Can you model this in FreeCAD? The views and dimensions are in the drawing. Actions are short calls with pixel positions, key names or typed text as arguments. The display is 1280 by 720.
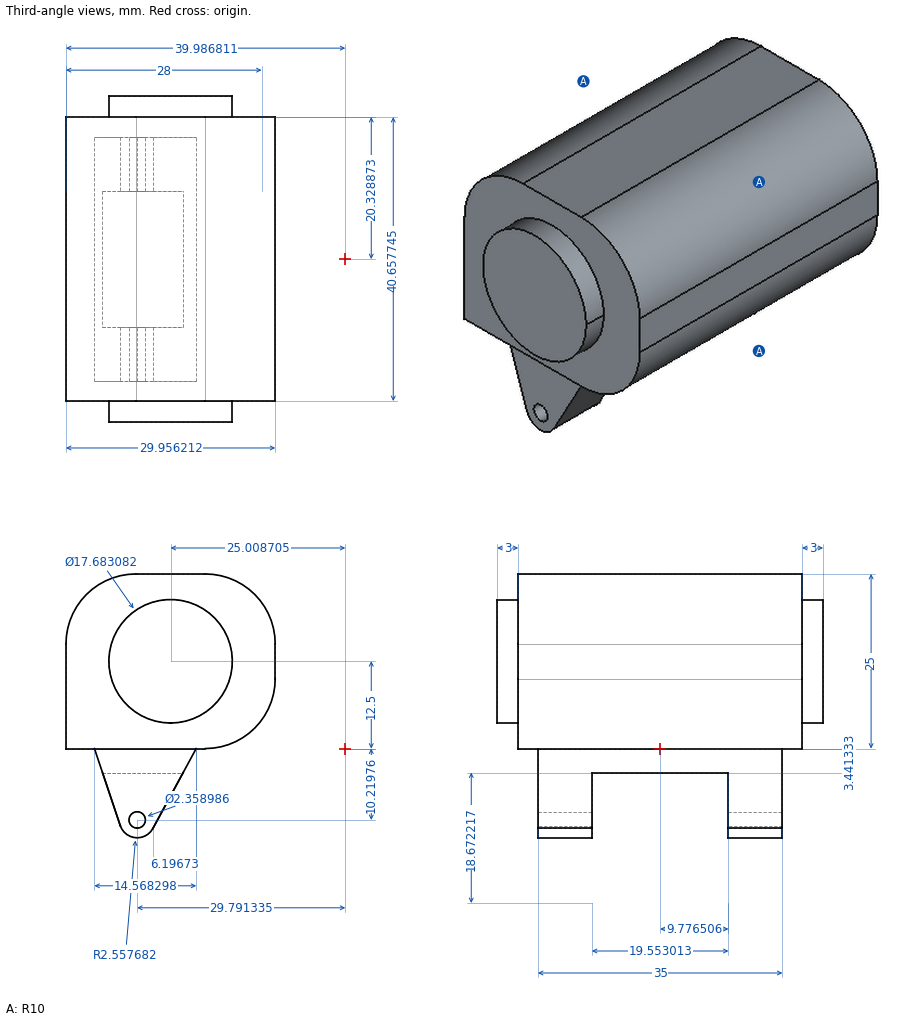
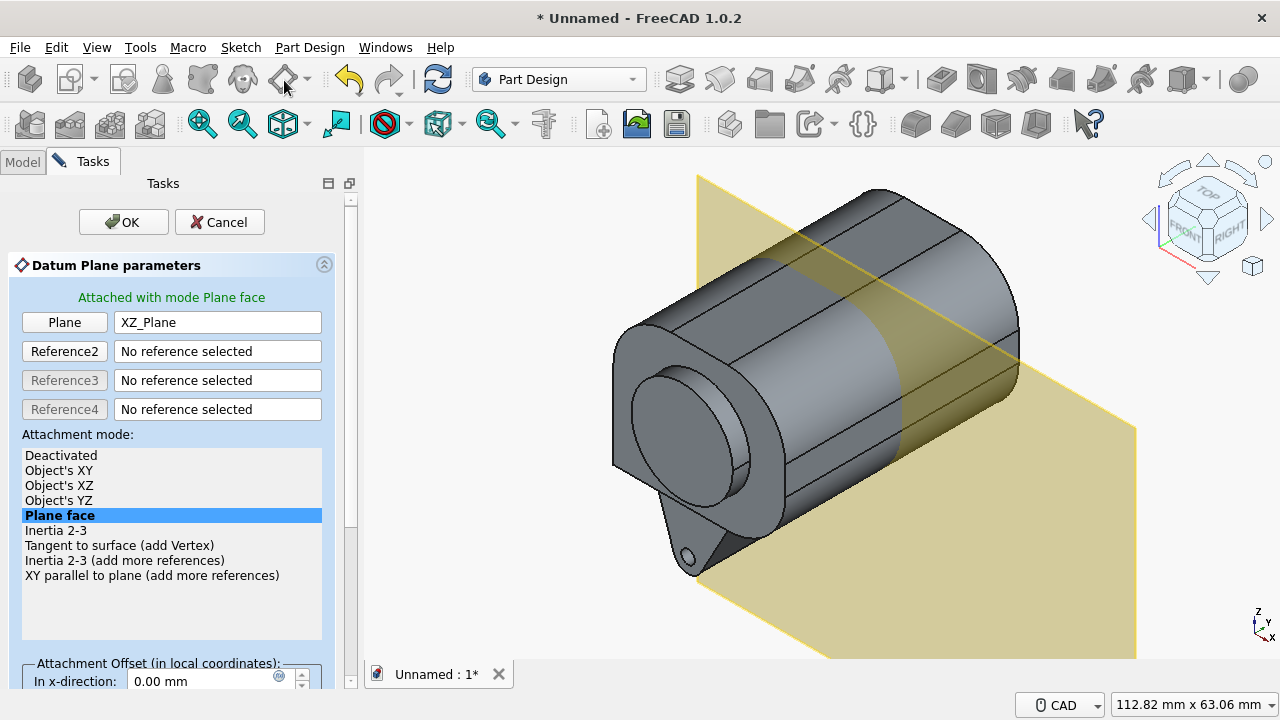
scroll(351, 440, down, 3)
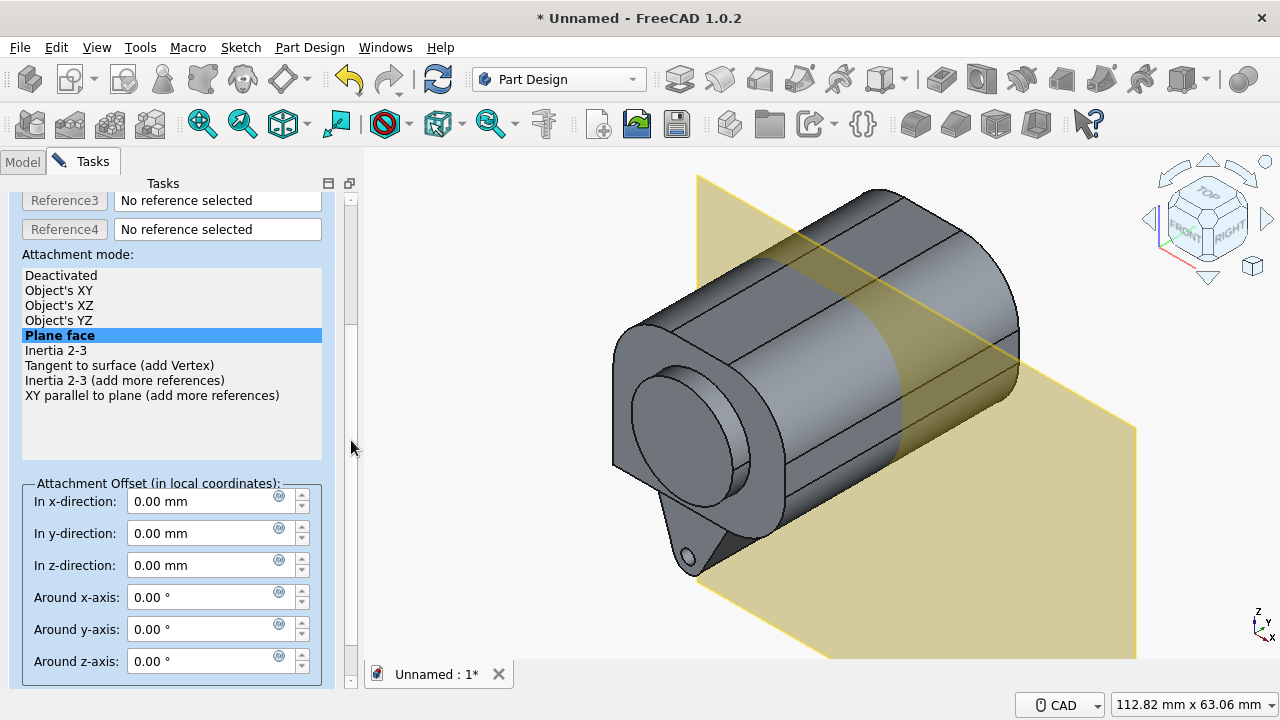
triple_click(210, 565)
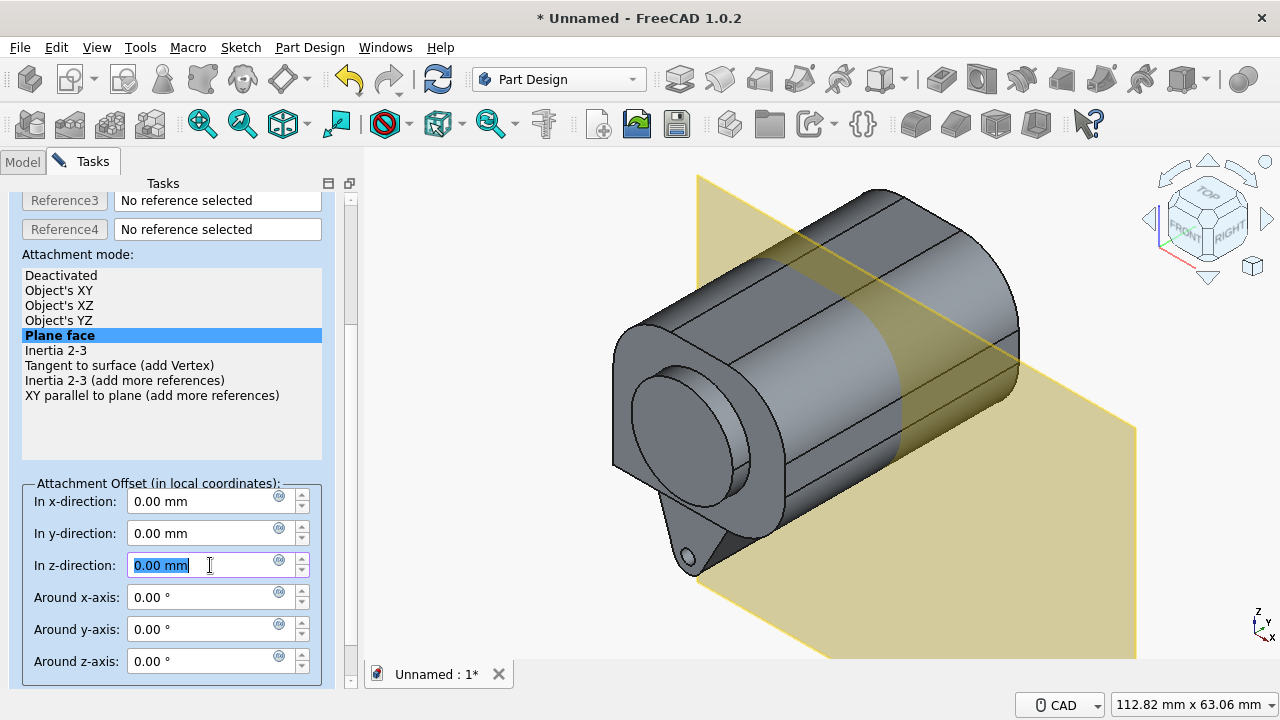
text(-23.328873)
key(Tab)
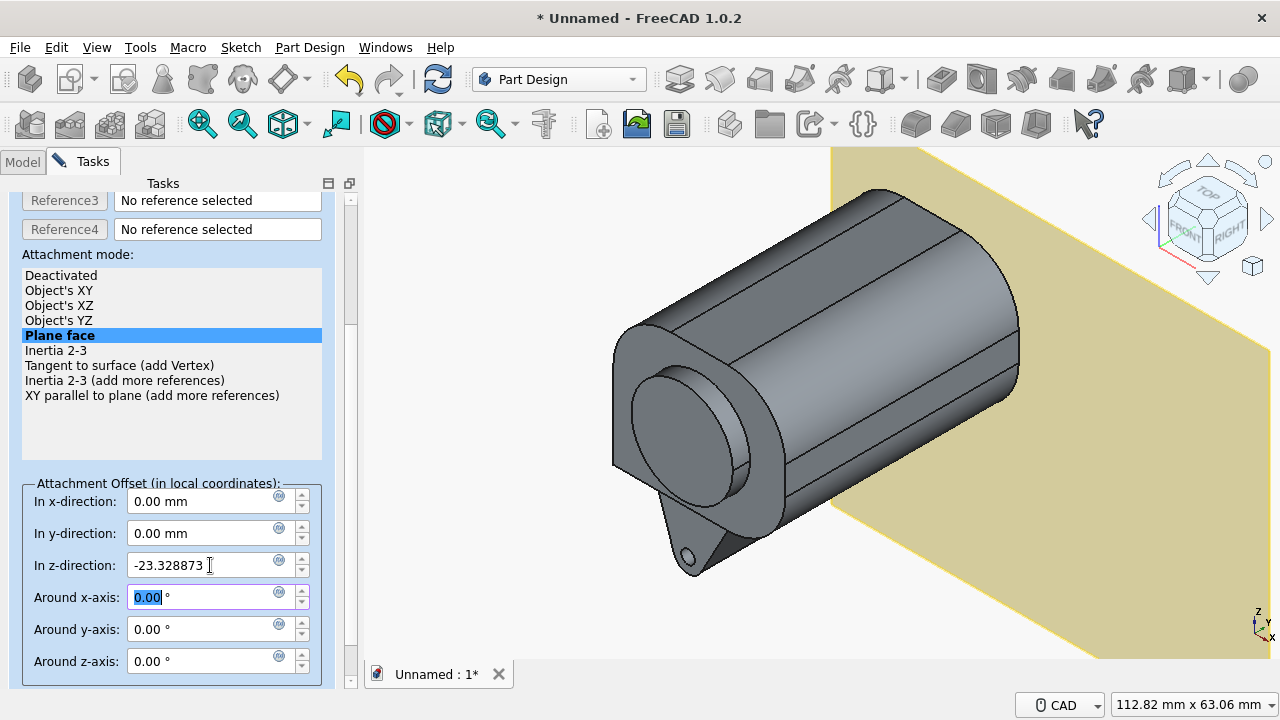
scroll(351, 440, up, 4)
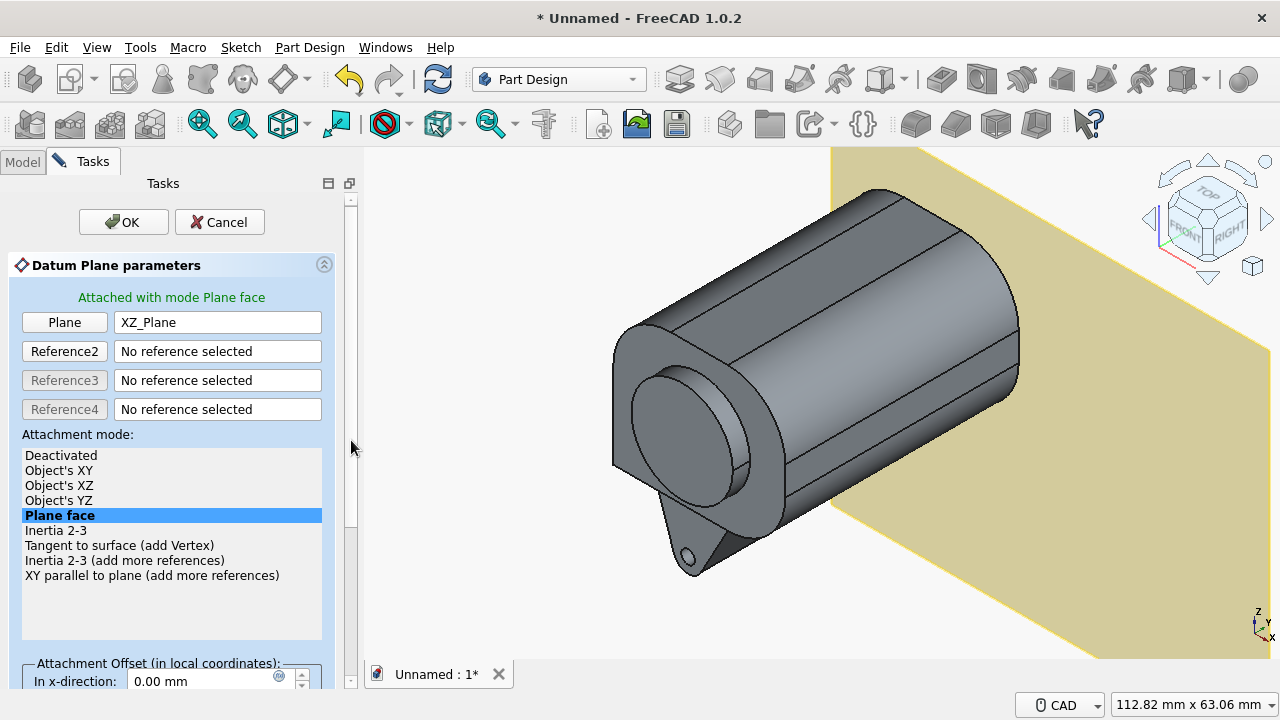
click(124, 222)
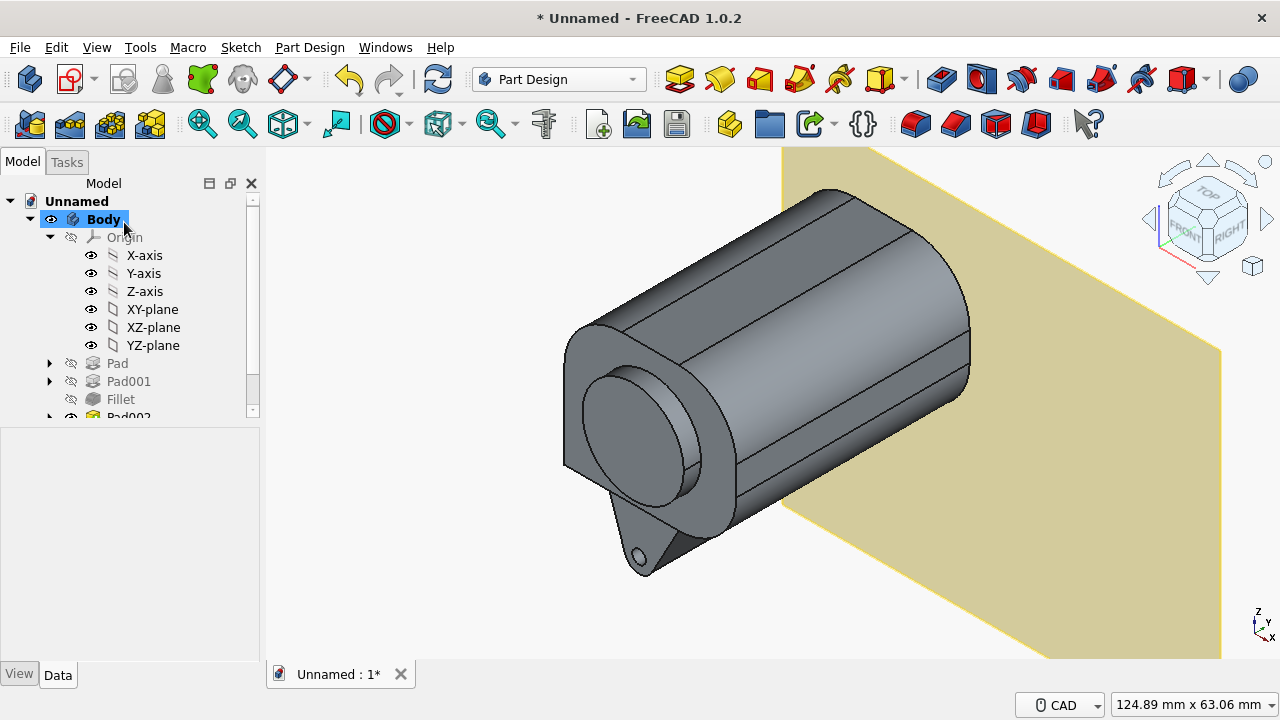
scroll(100, 305, down, 3)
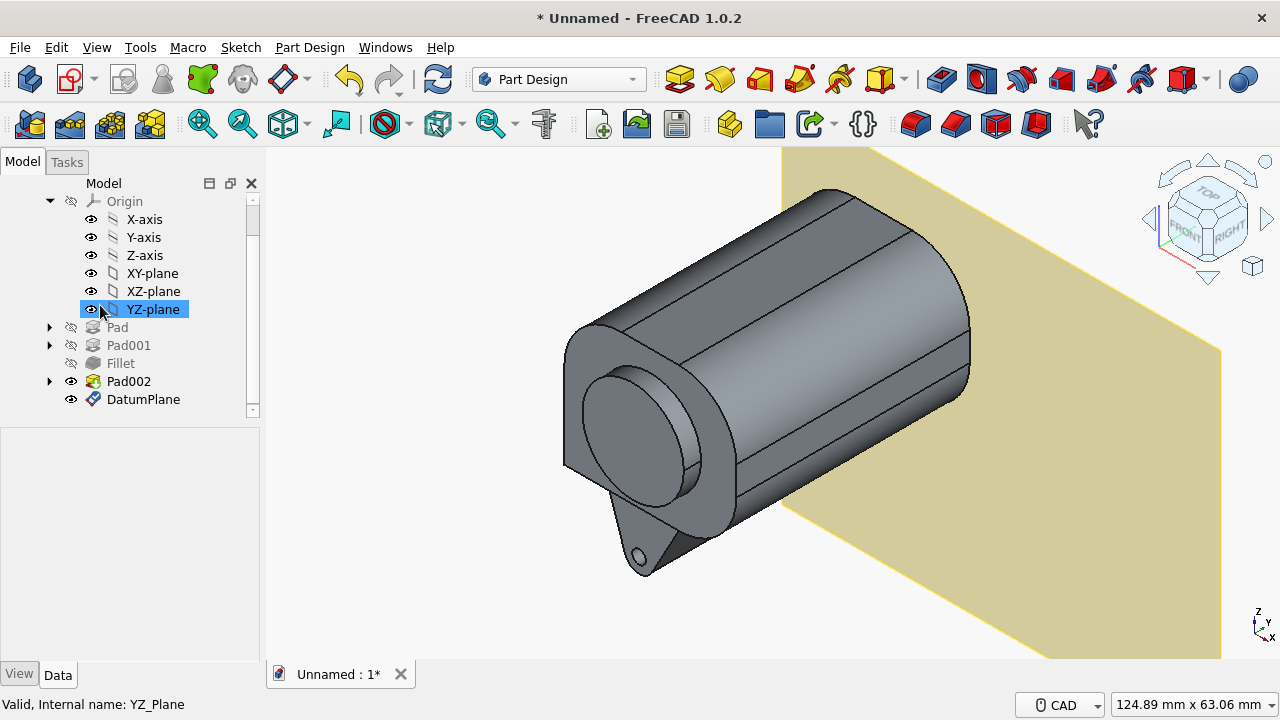
click(116, 399)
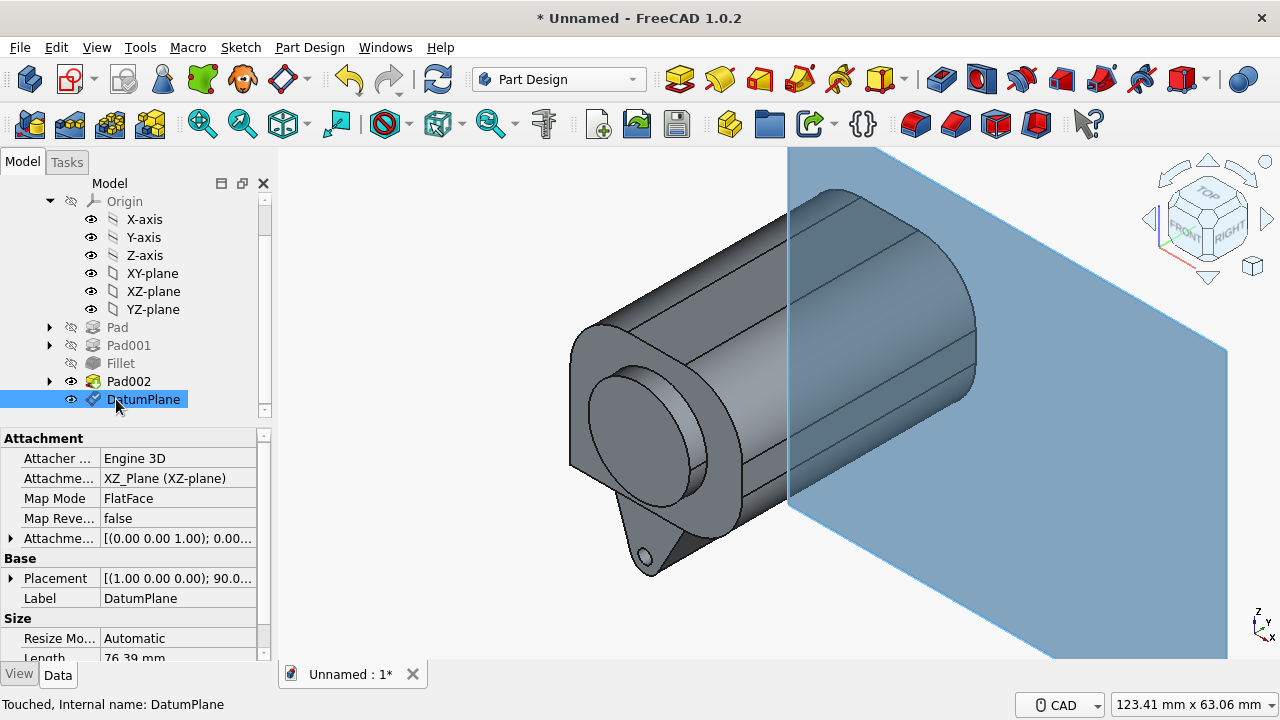
click(70, 80)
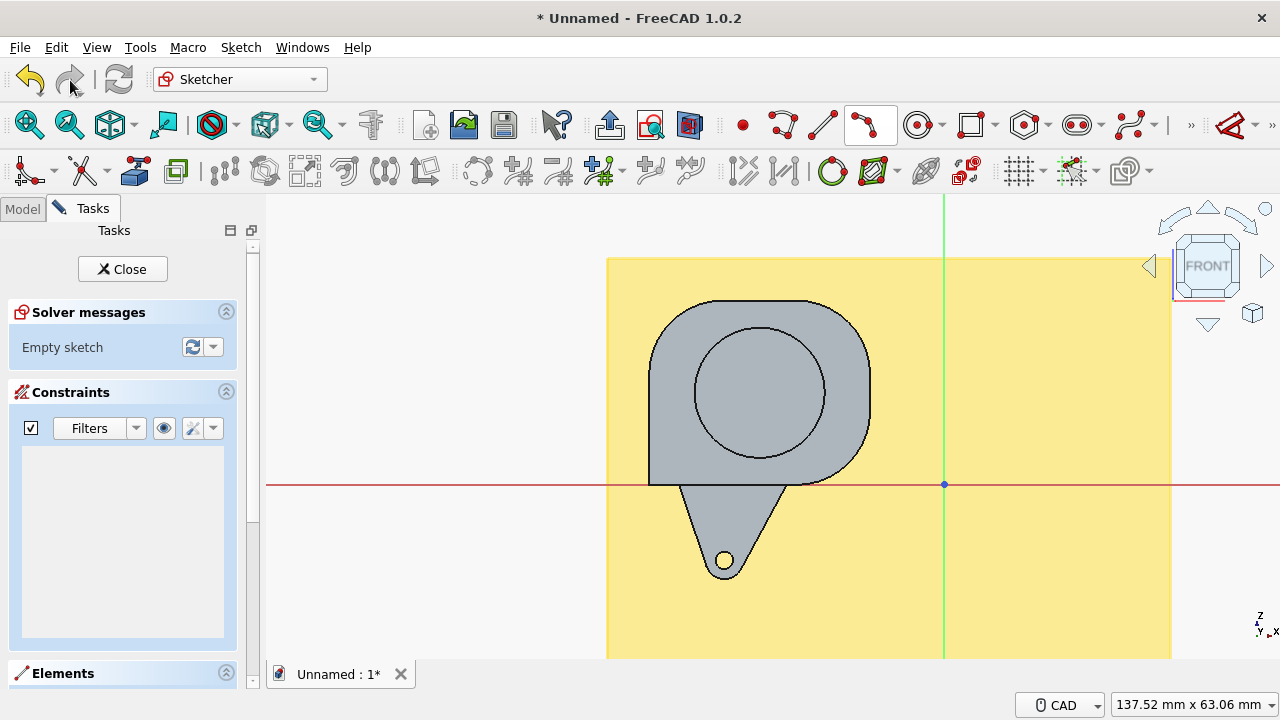
click(690, 126)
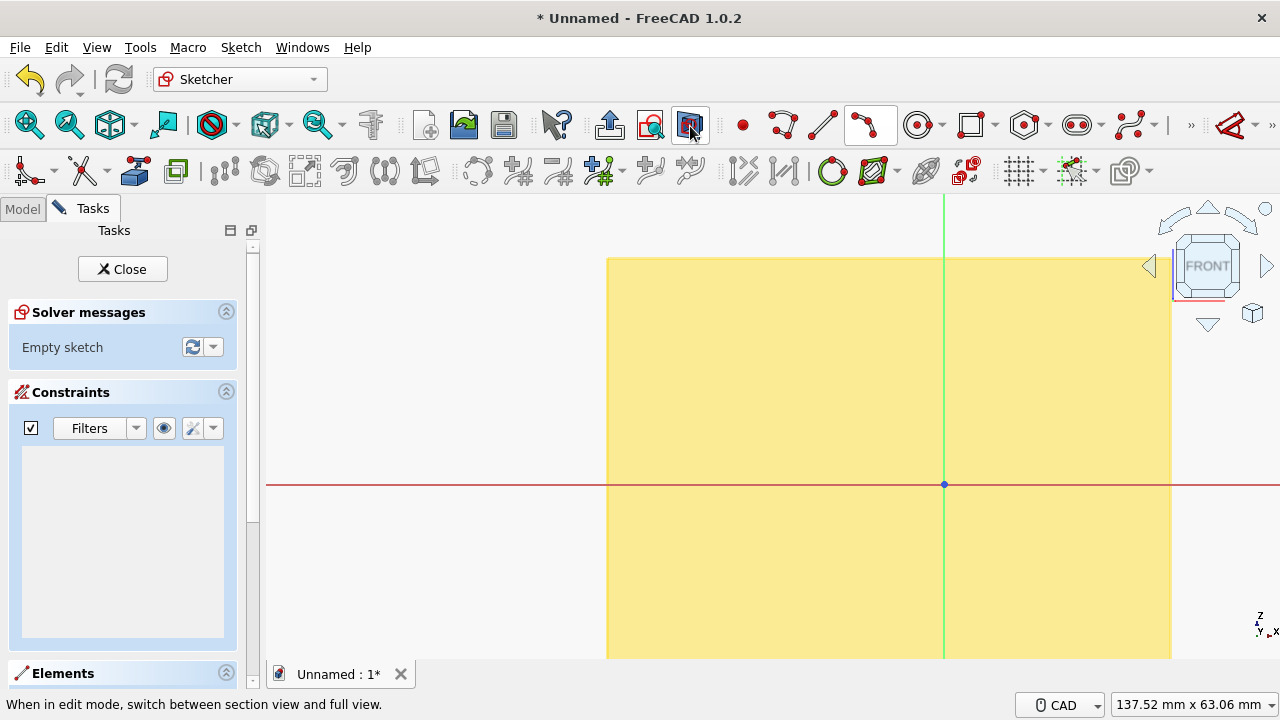
scroll(959, 382, up, 3)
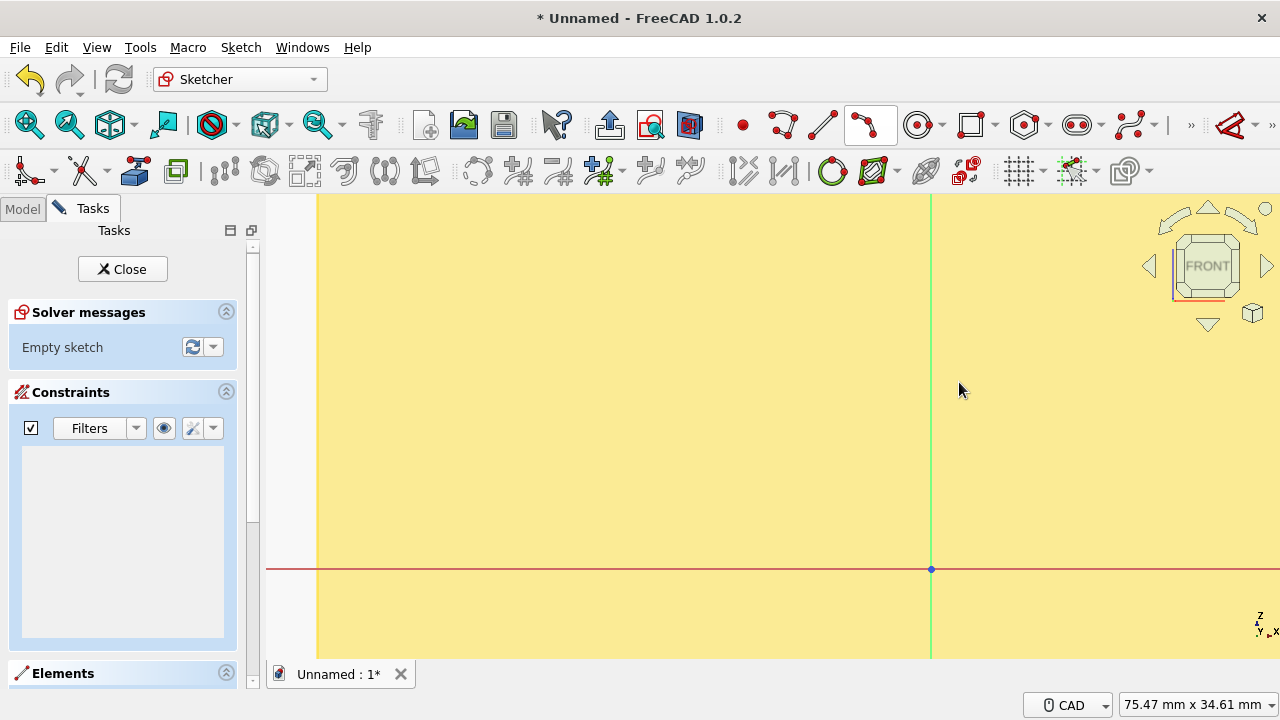
click(918, 126)